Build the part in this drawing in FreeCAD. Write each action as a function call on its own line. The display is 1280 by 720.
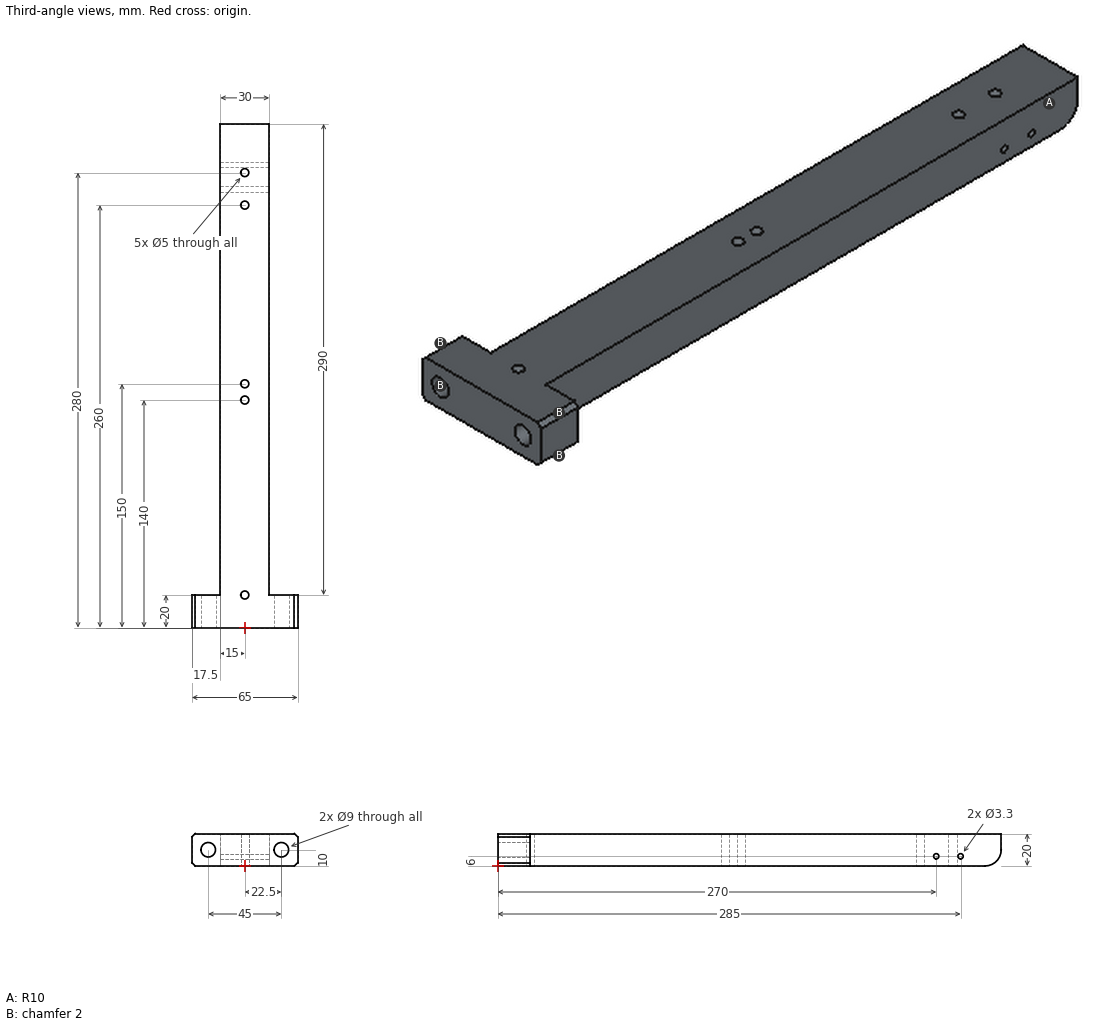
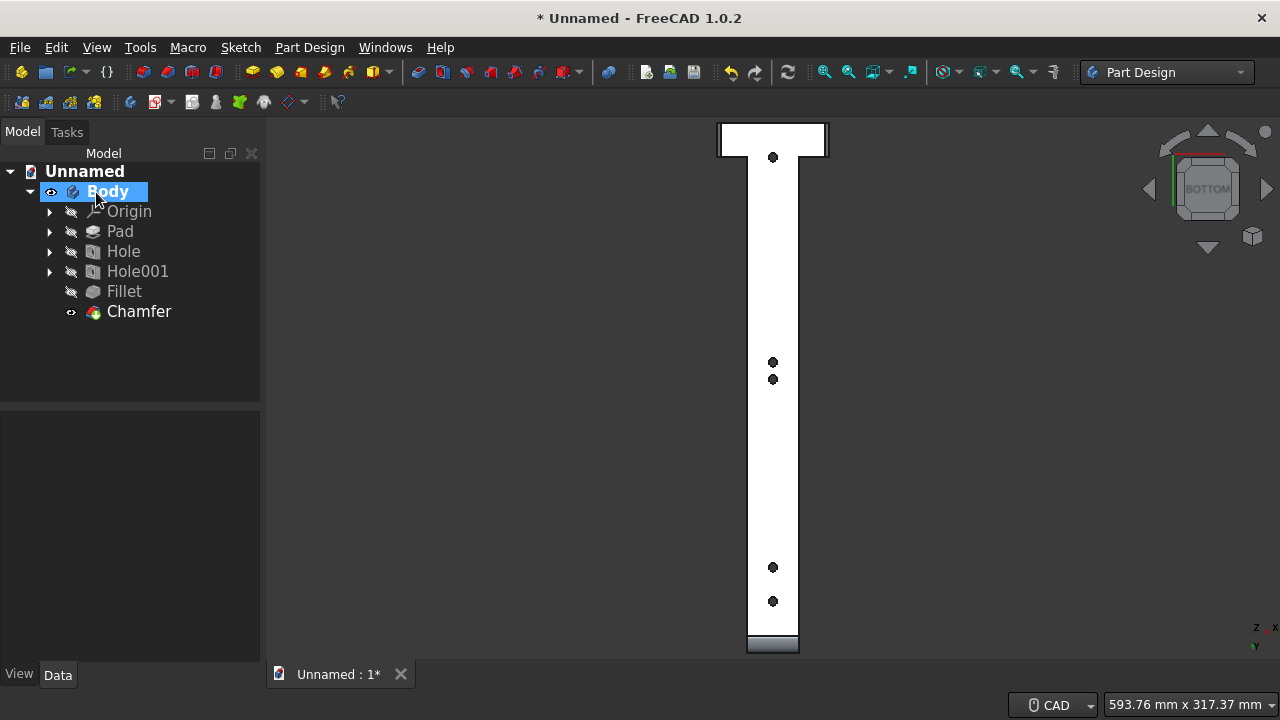
key(6)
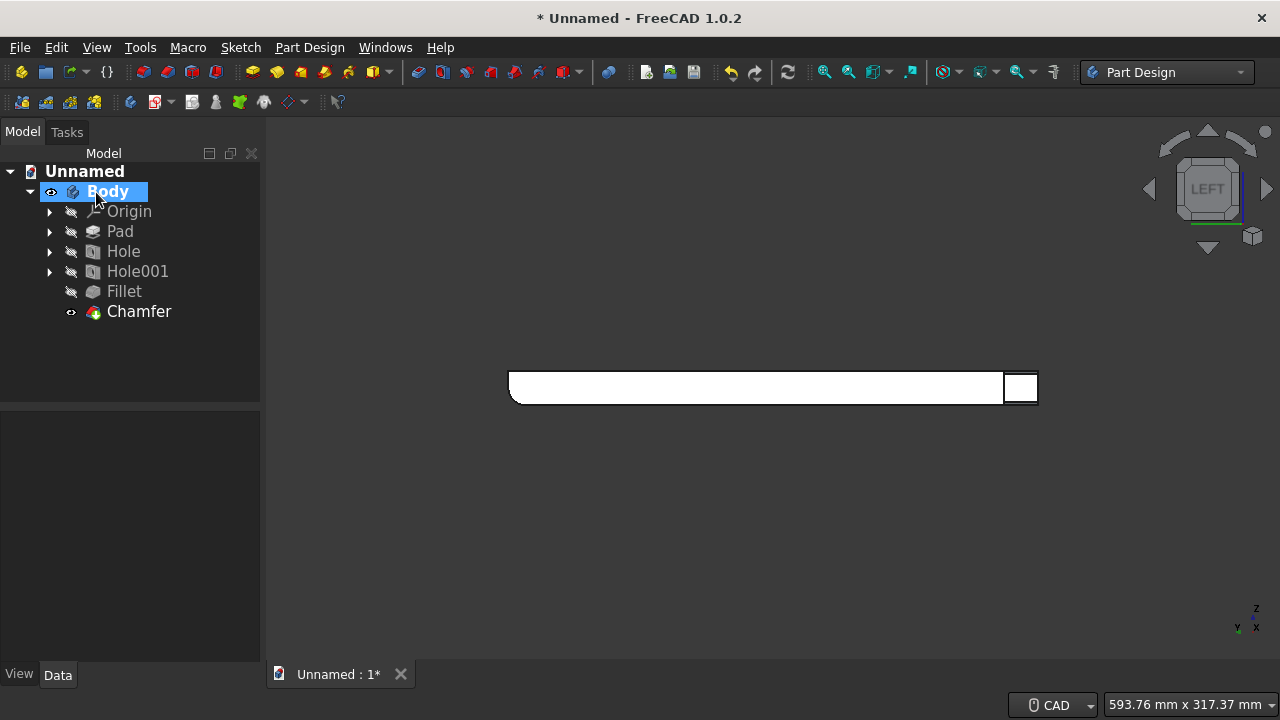
click(544, 387)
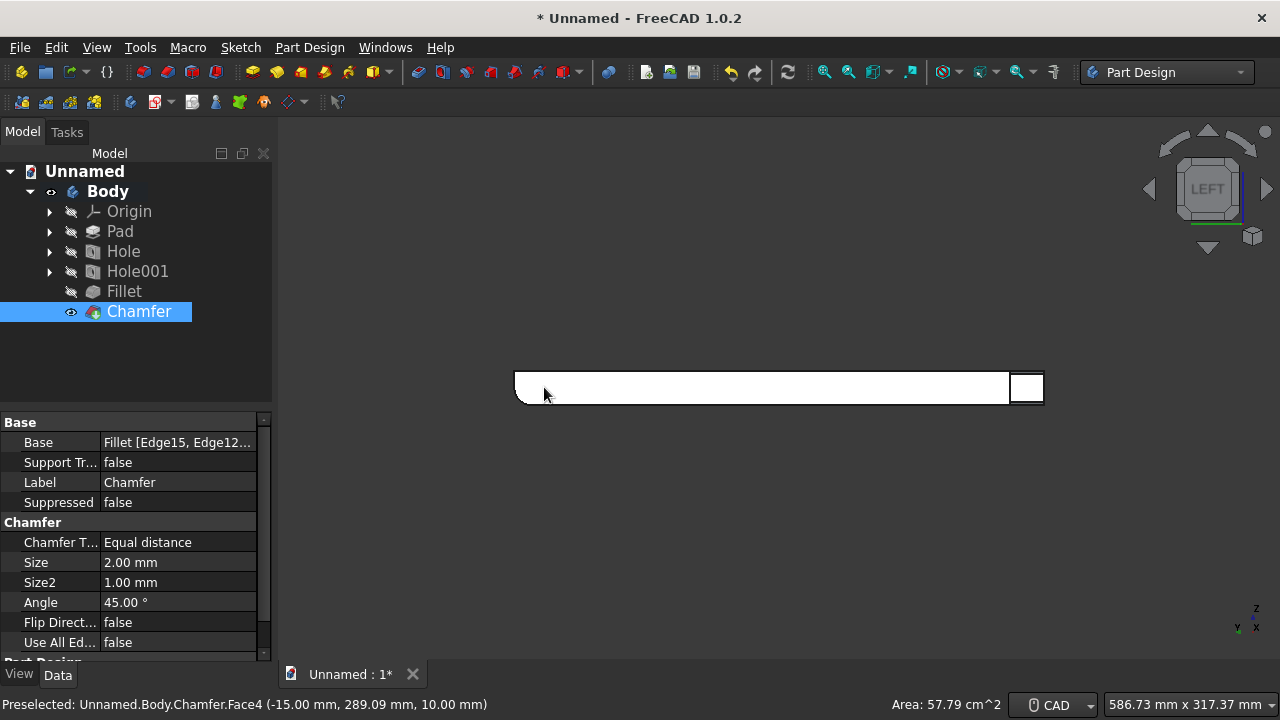
click(156, 102)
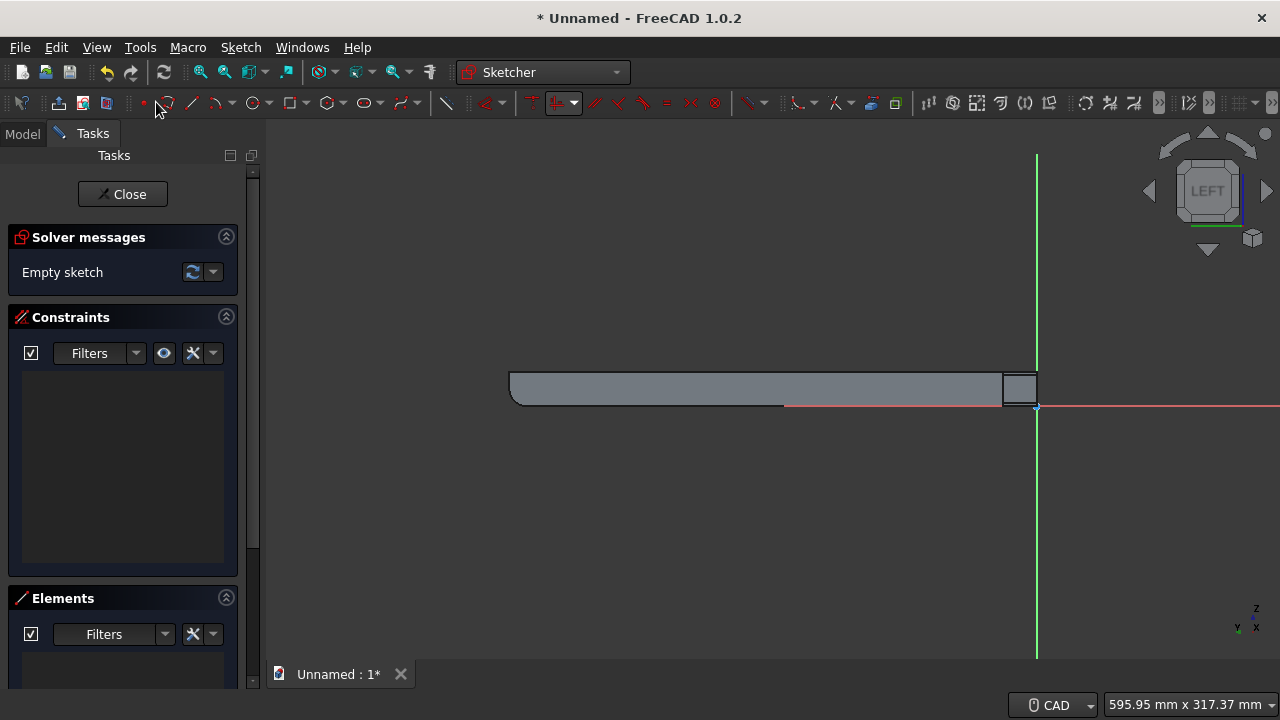
key(q)
key(s)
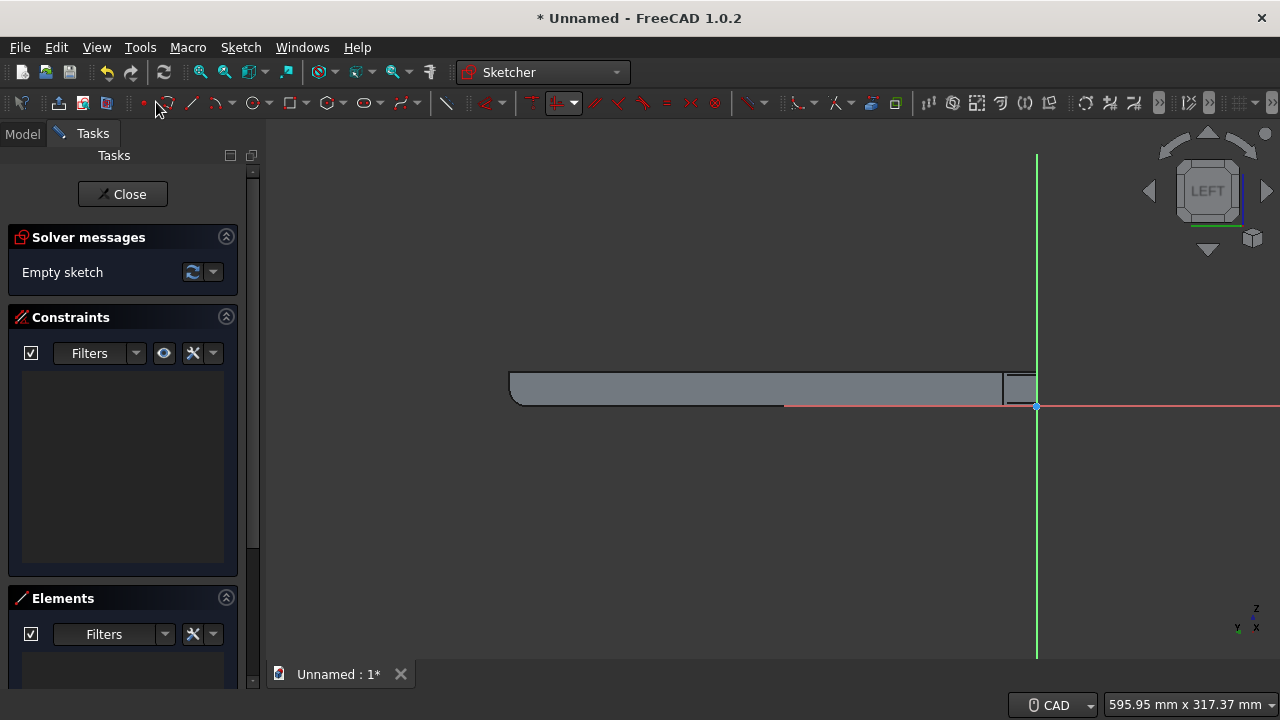
scroll(557, 396, up, 15)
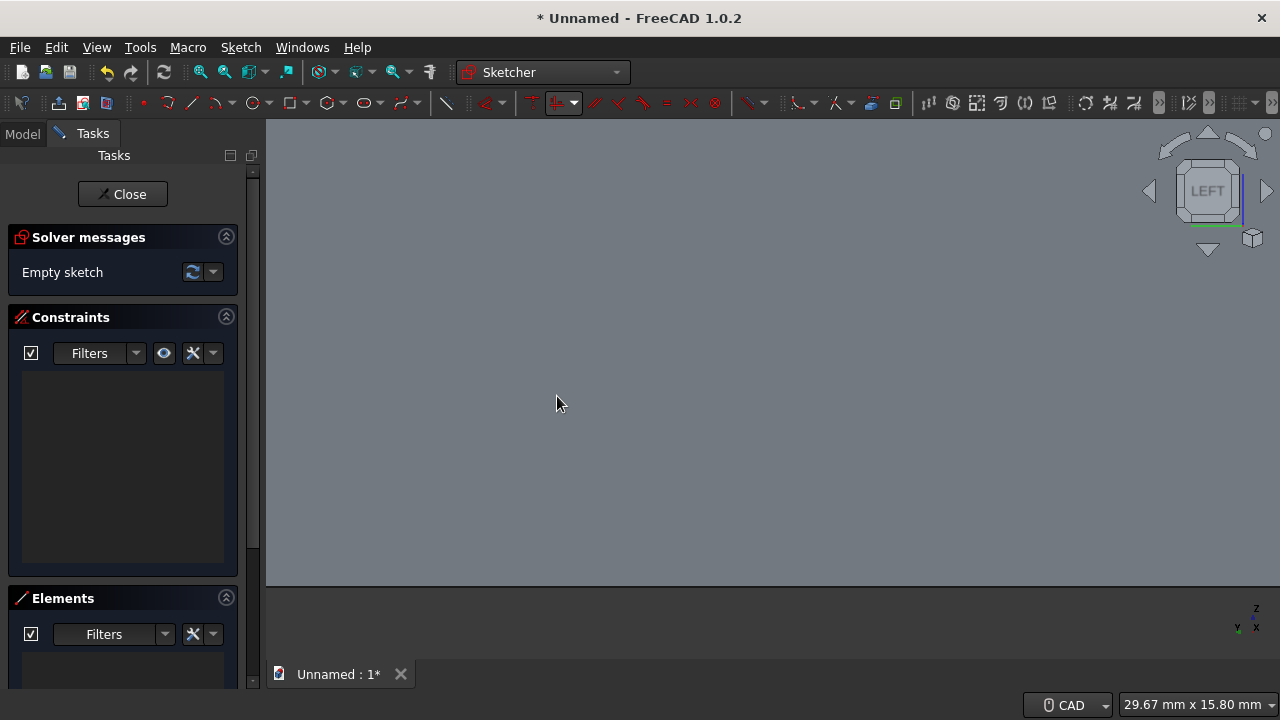
click(254, 104)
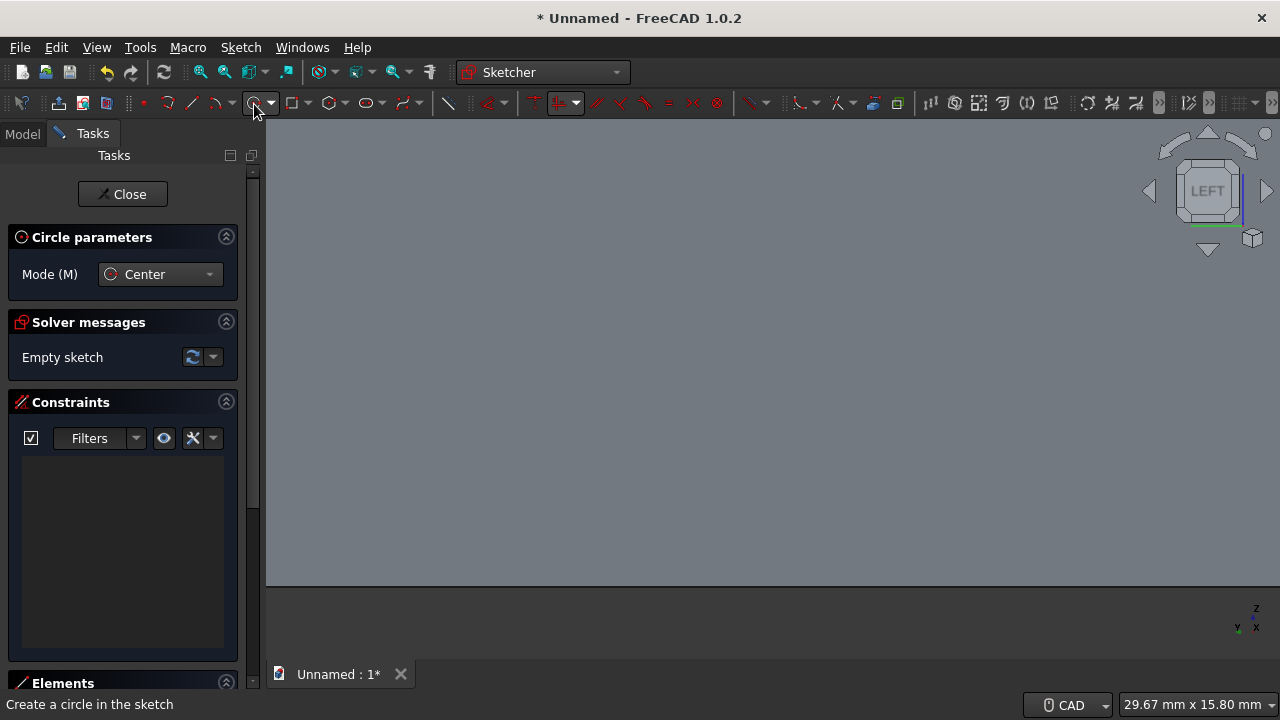
click(447, 382)
click(487, 342)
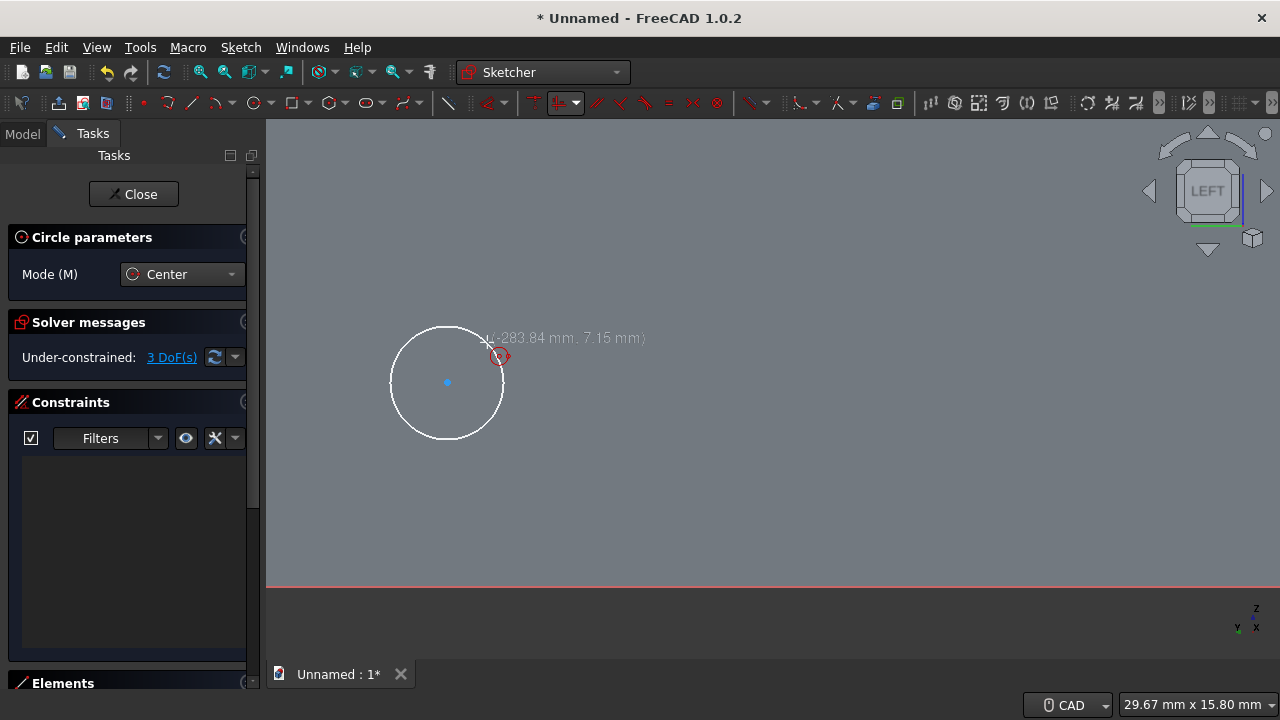
click(960, 382)
click(1000, 342)
key(Escape)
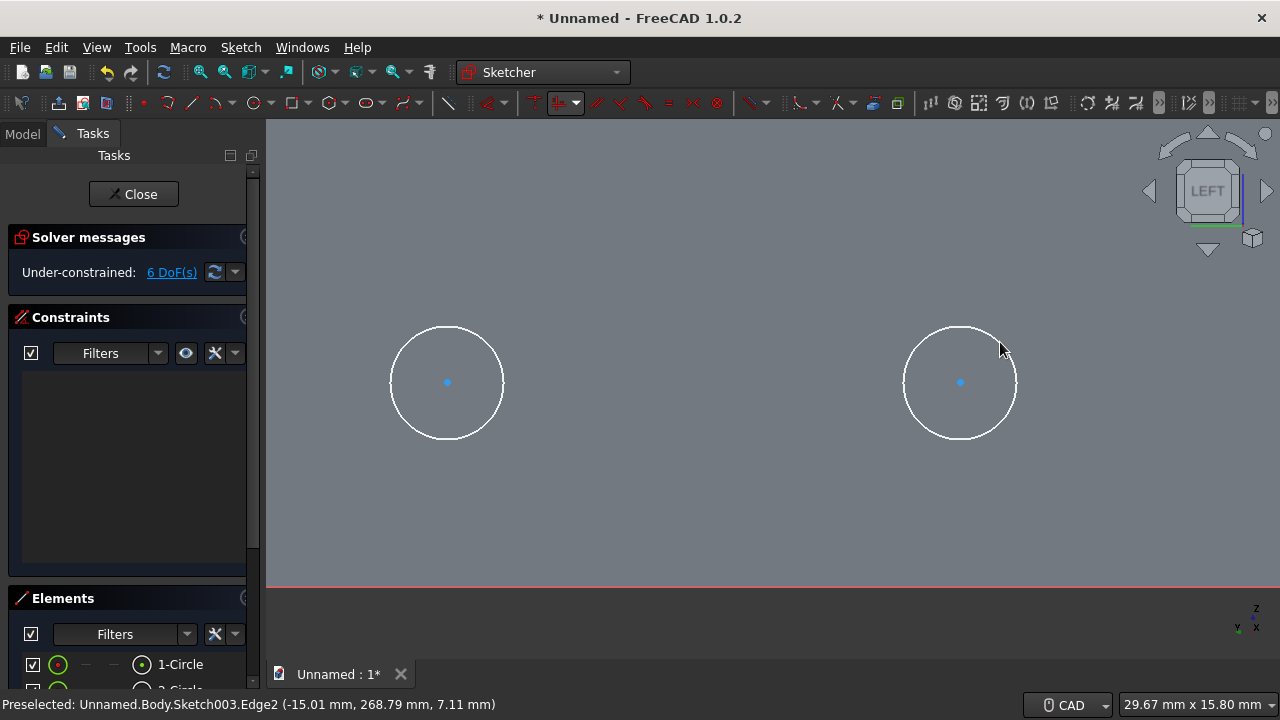
click(487, 343)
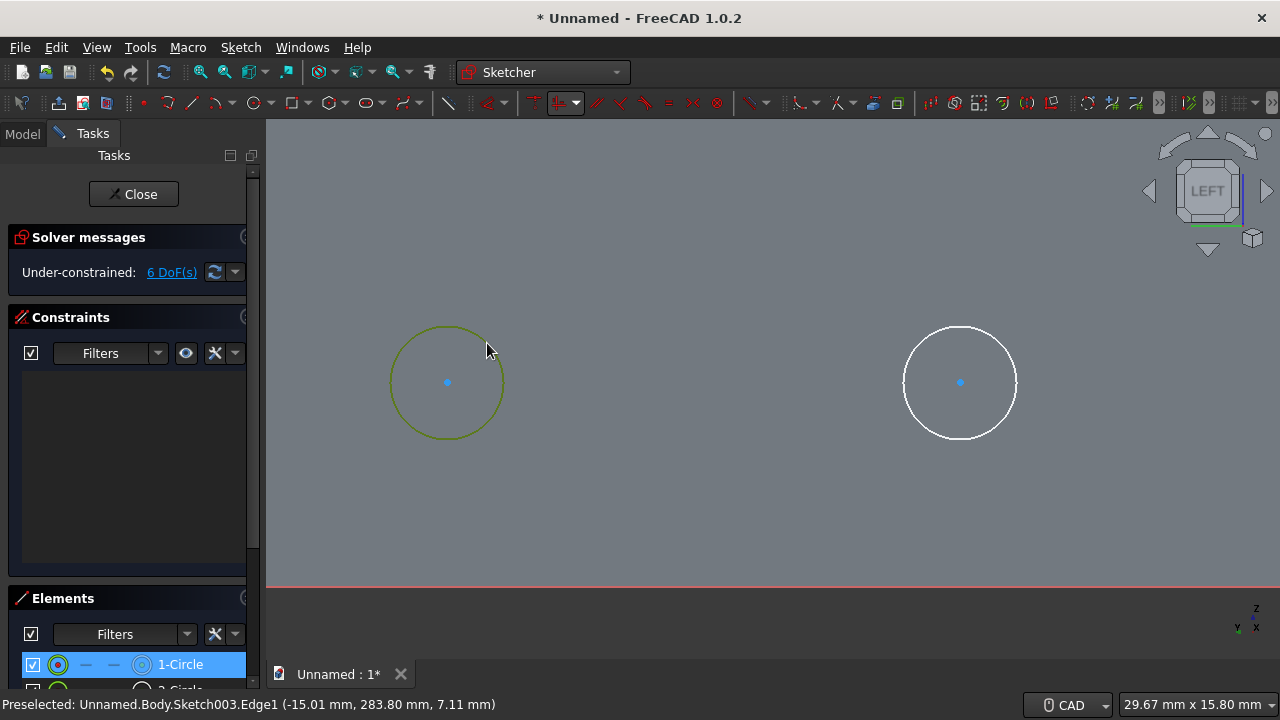
click(1000, 343)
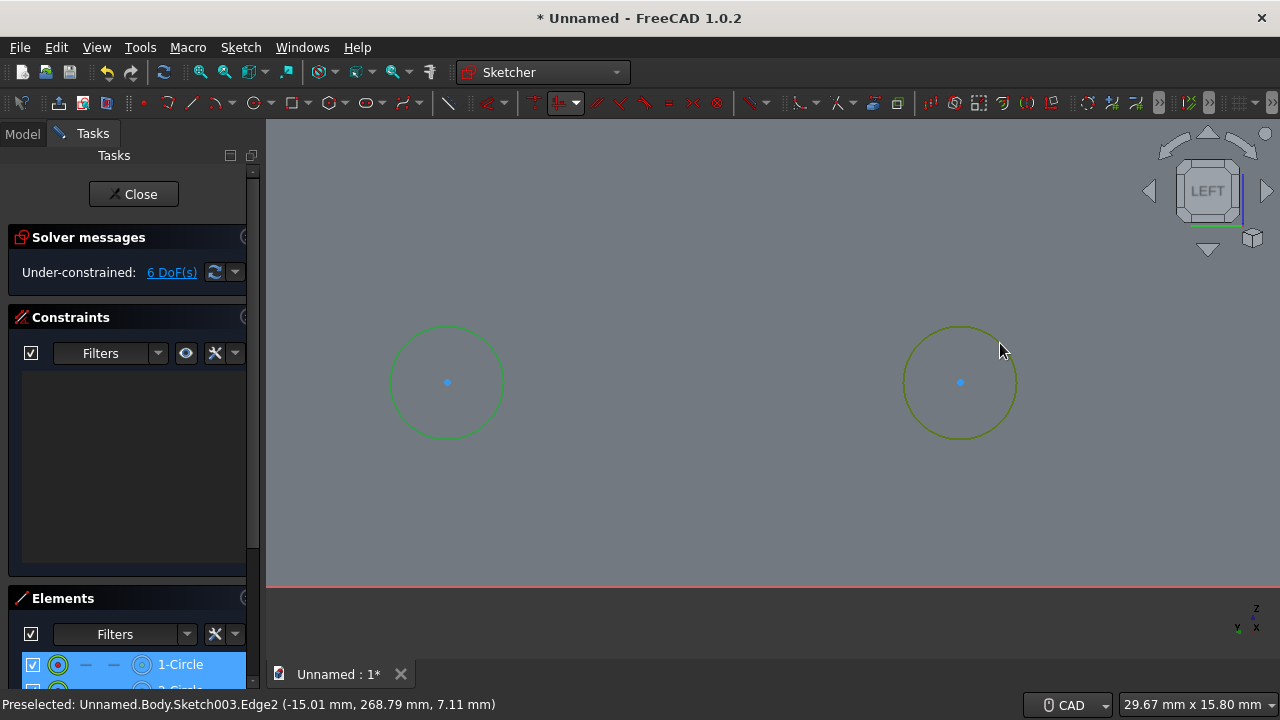
click(670, 104)